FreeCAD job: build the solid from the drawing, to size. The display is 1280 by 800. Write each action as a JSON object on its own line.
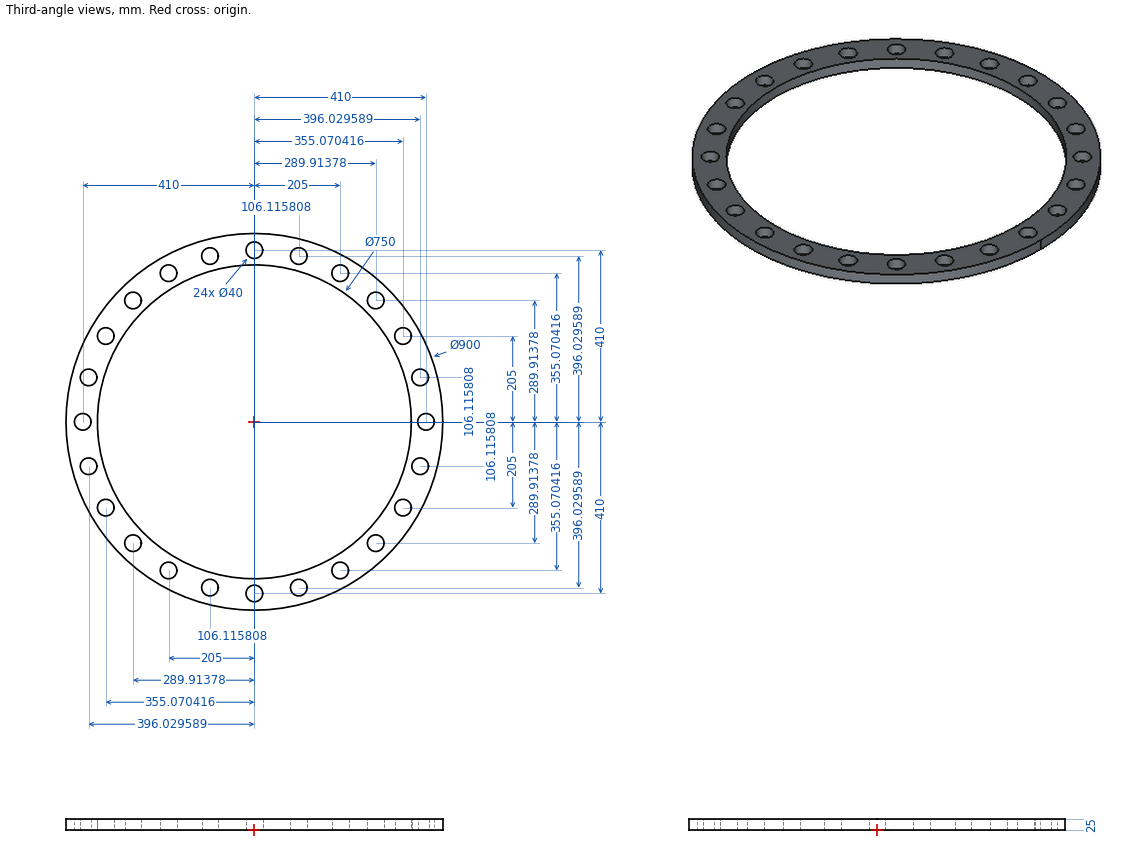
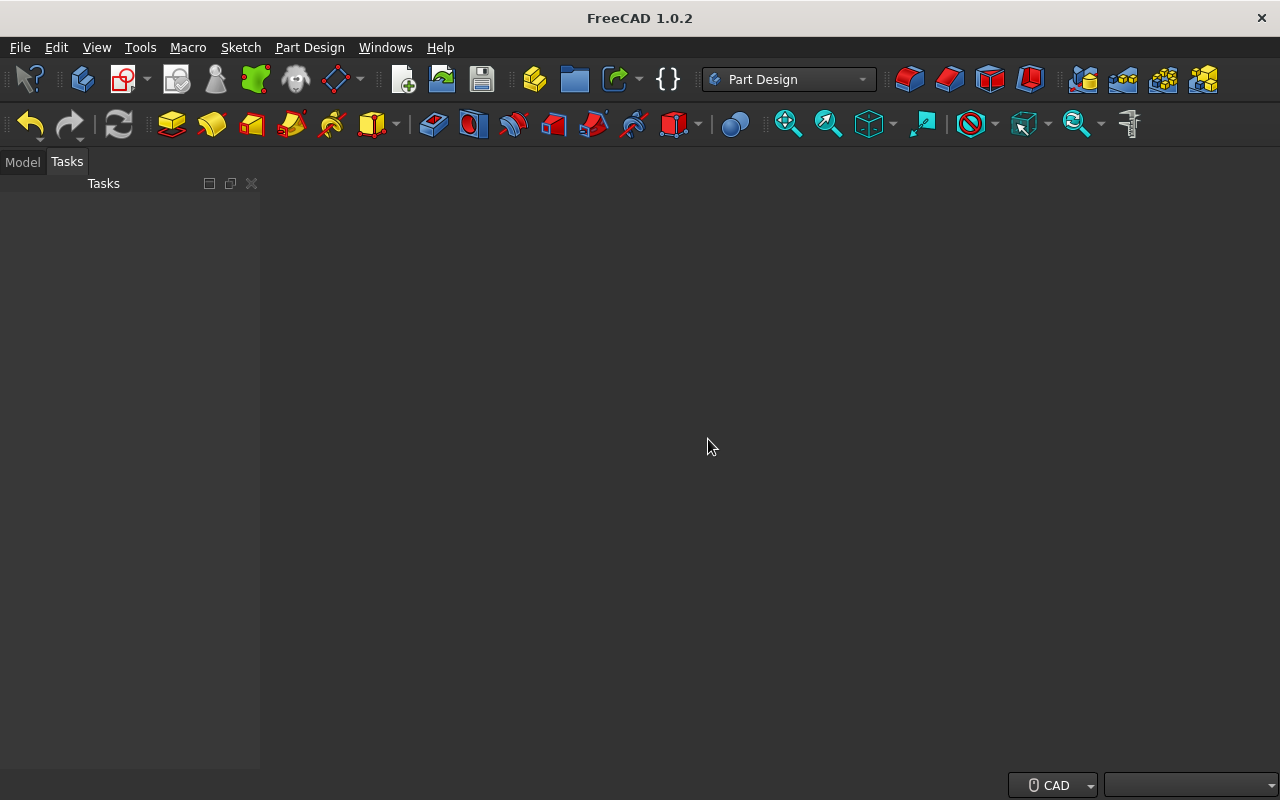
{"action": "left_click", "coordinate": [402, 80]}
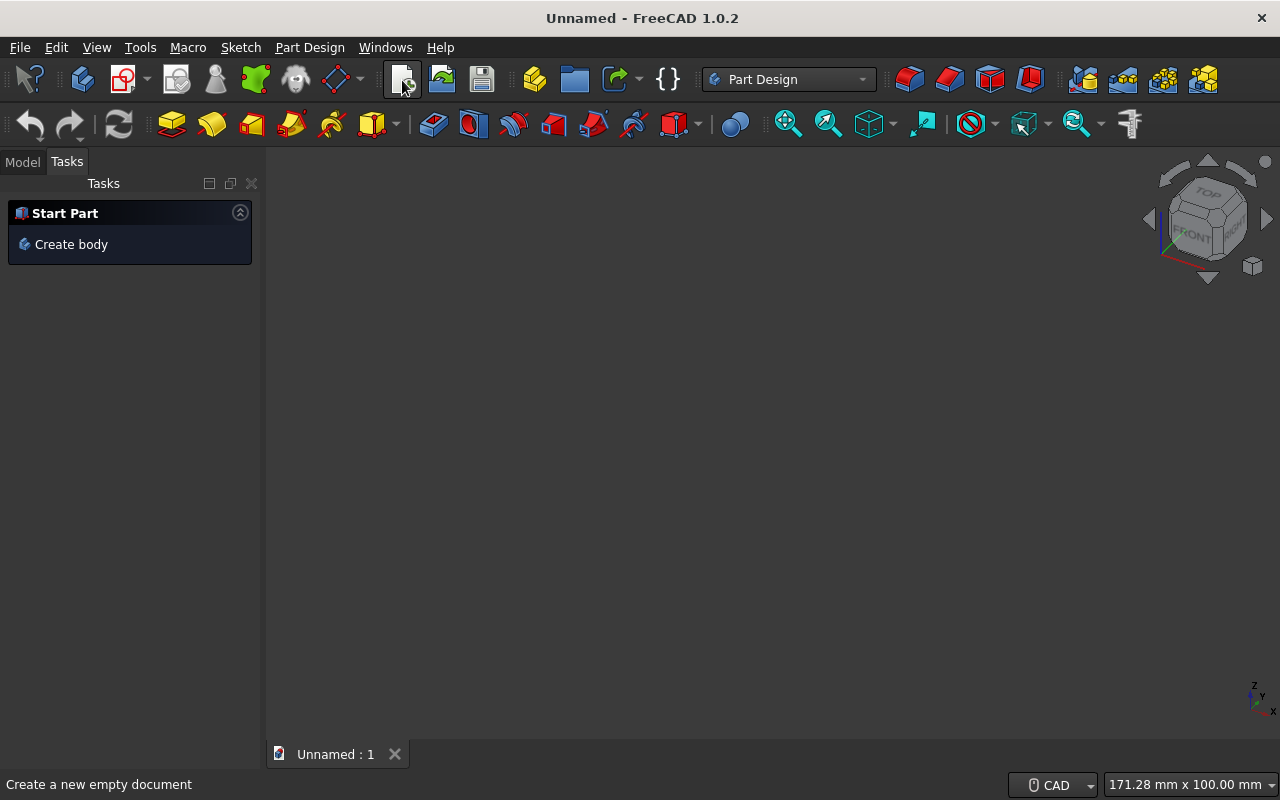
{"action": "left_click", "coordinate": [124, 80]}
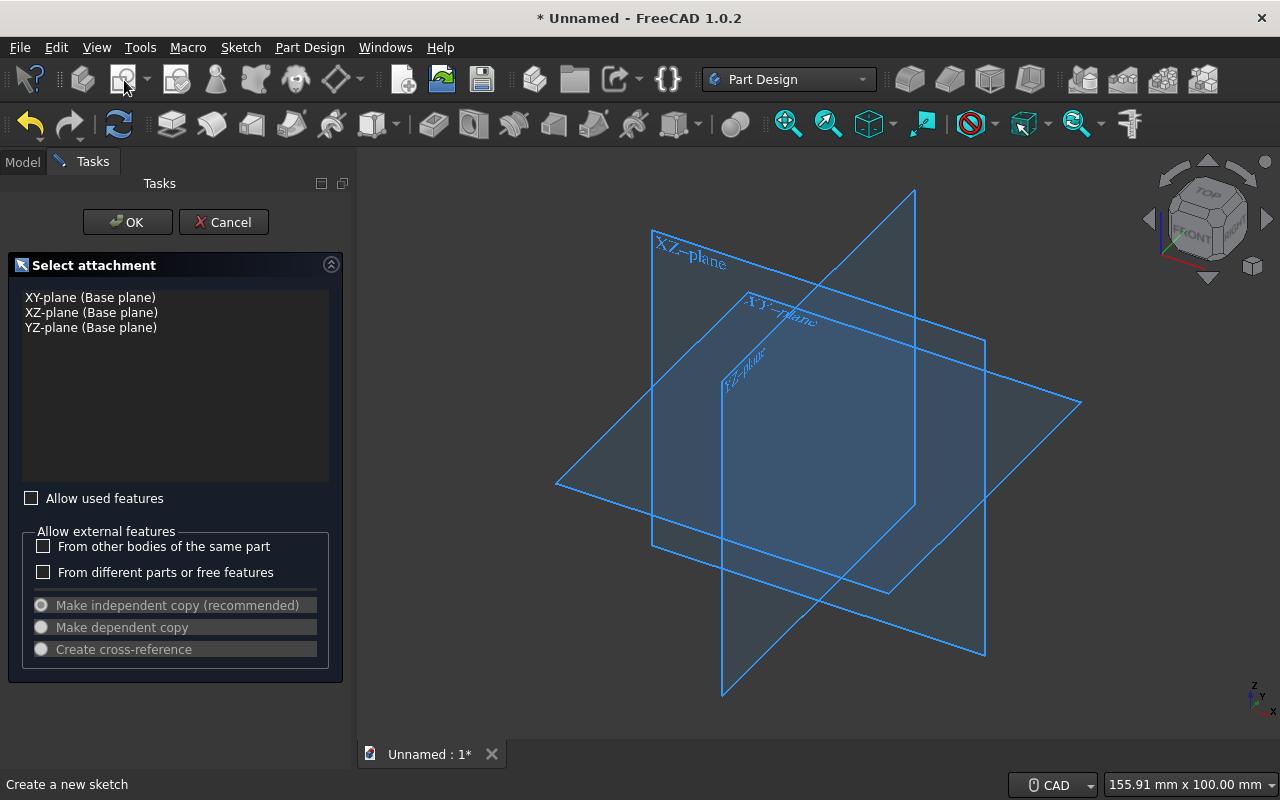
{"action": "left_click", "coordinate": [82, 298]}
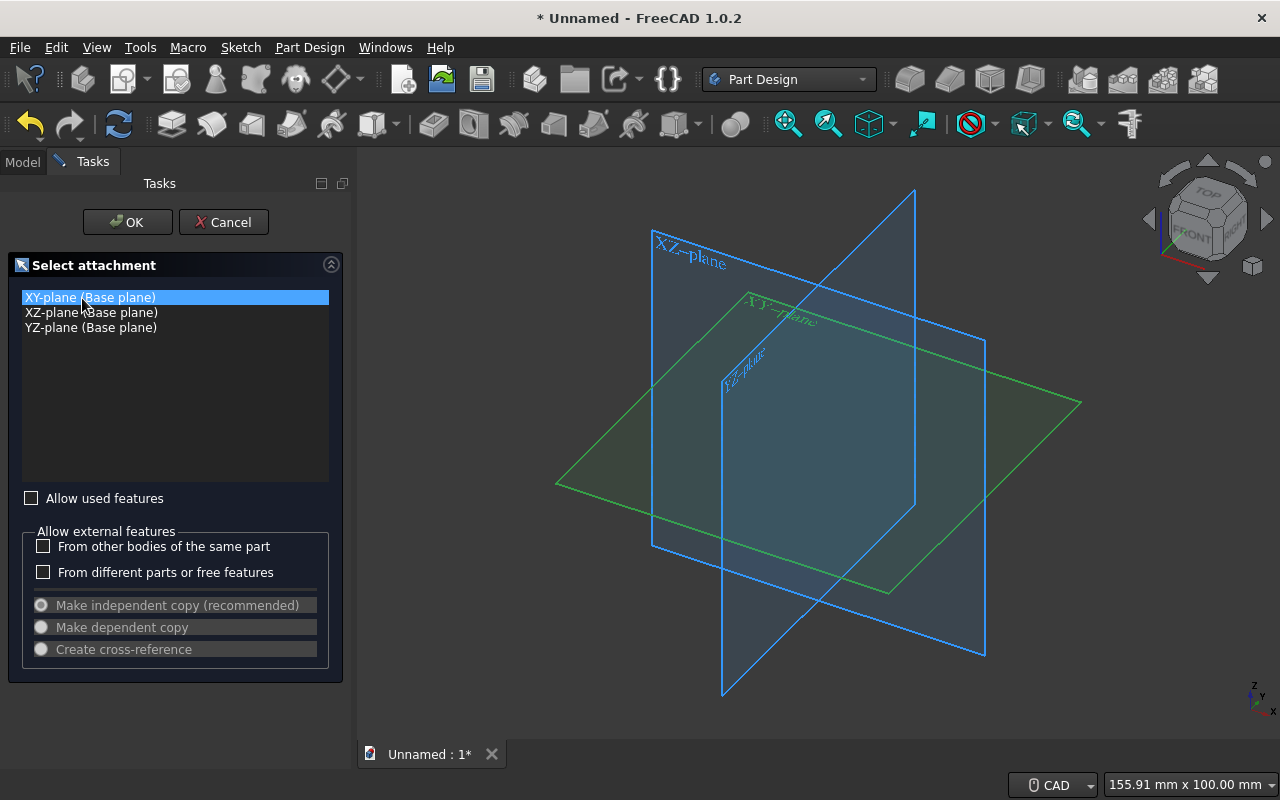
{"action": "left_click", "coordinate": [128, 222]}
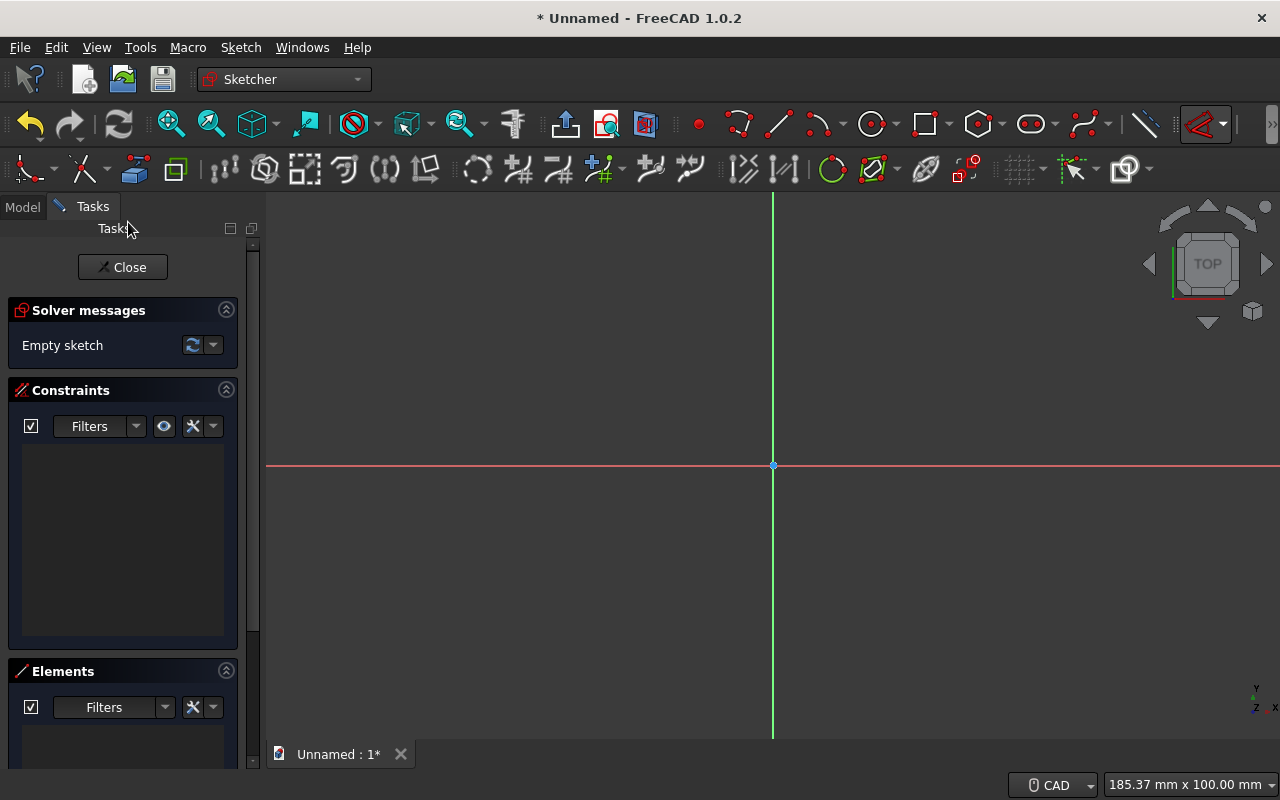
{"action": "scroll", "coordinate": [699, 466], "scroll_direction": "down", "scroll_amount": 13}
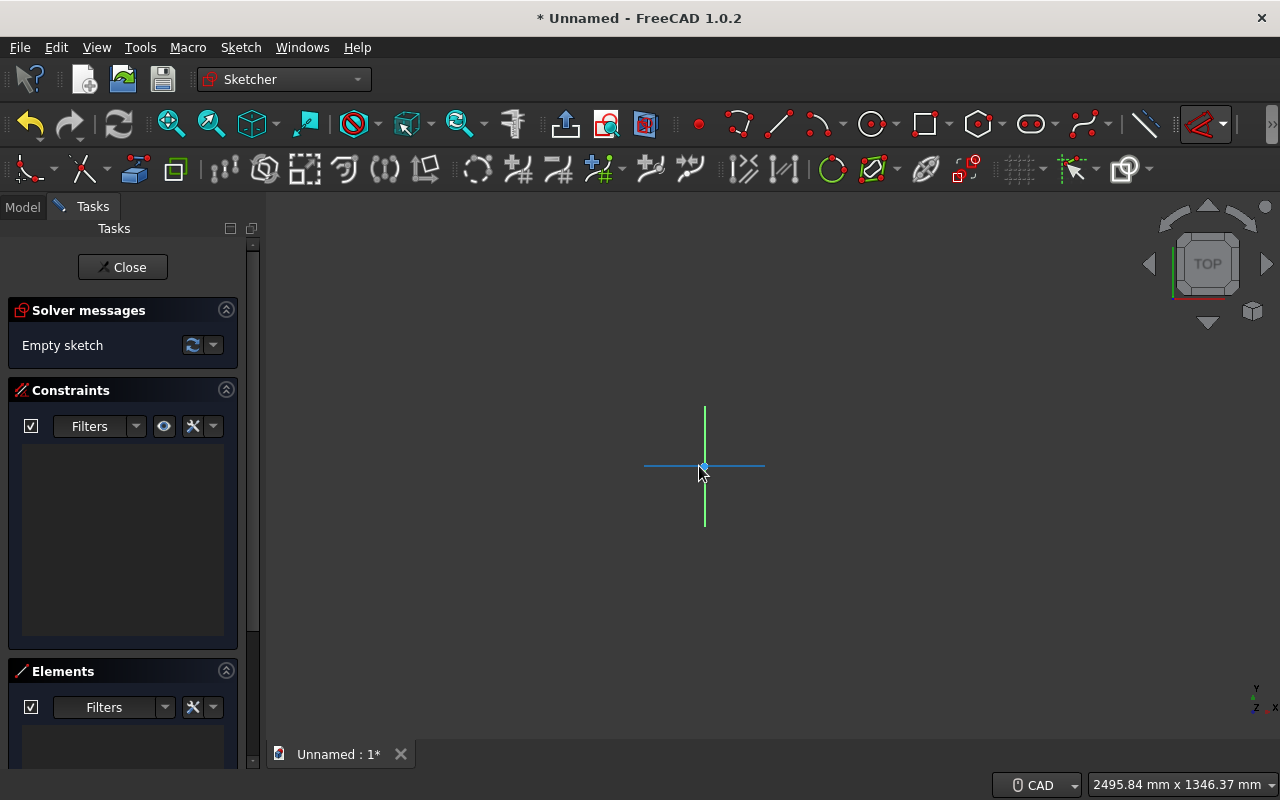
{"action": "left_click", "coordinate": [872, 124]}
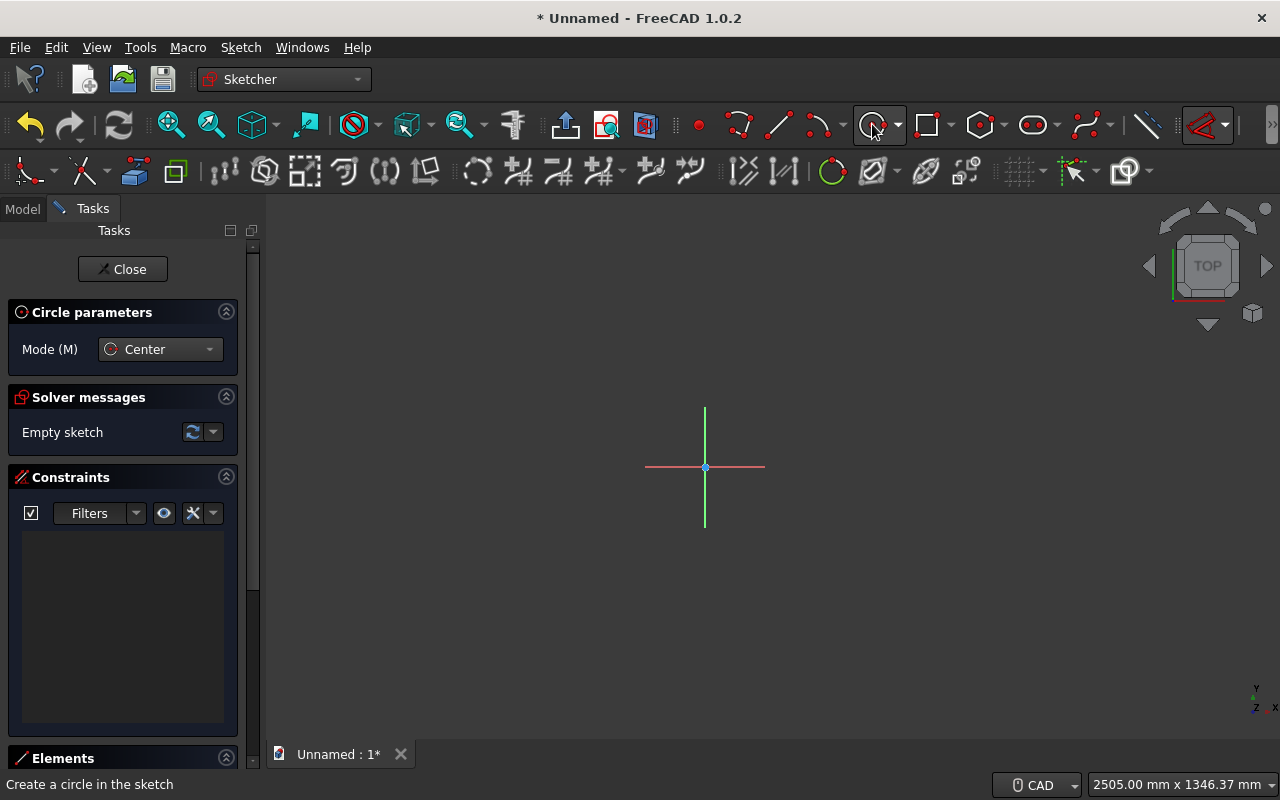
{"action": "left_click", "coordinate": [705, 467]}
{"action": "mouse_move", "coordinate": [834, 339]}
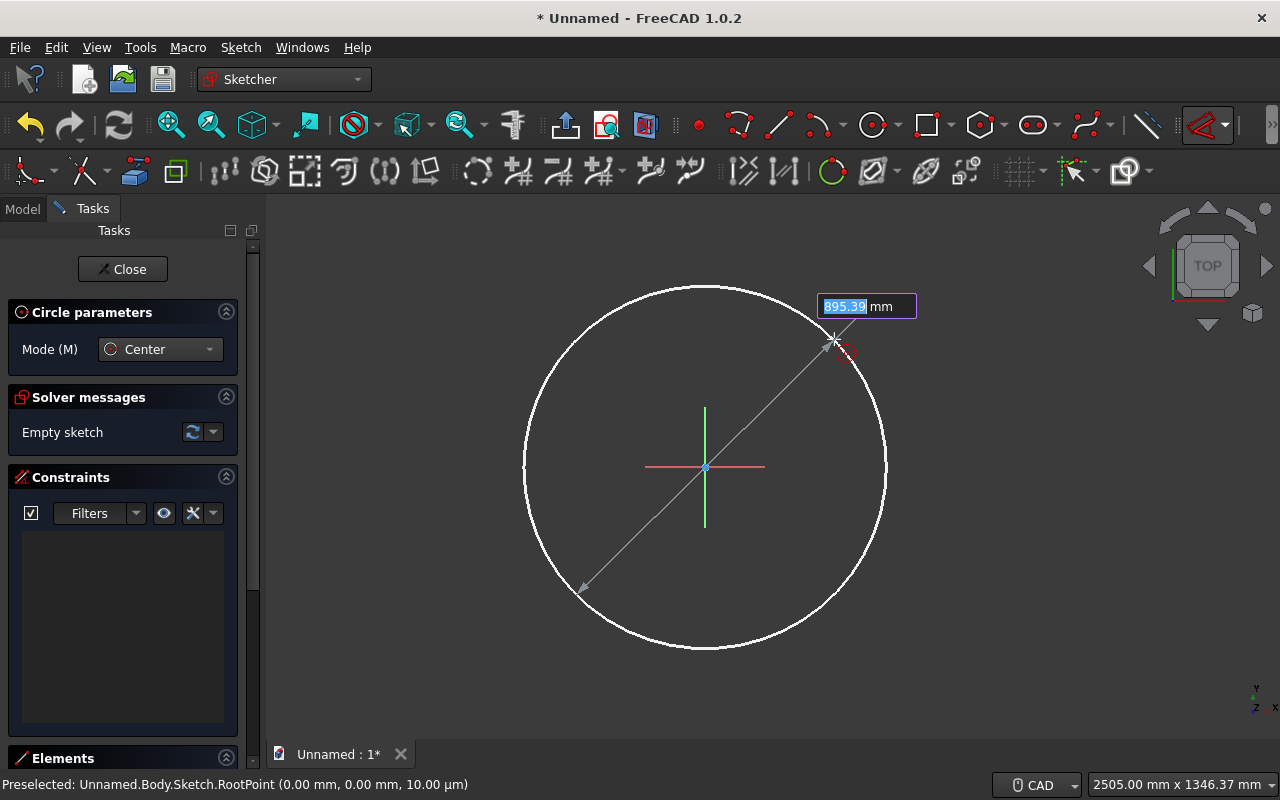
{"action": "type", "text": "900"}
{"action": "key", "text": "Return"}
{"action": "key", "text": "Escape"}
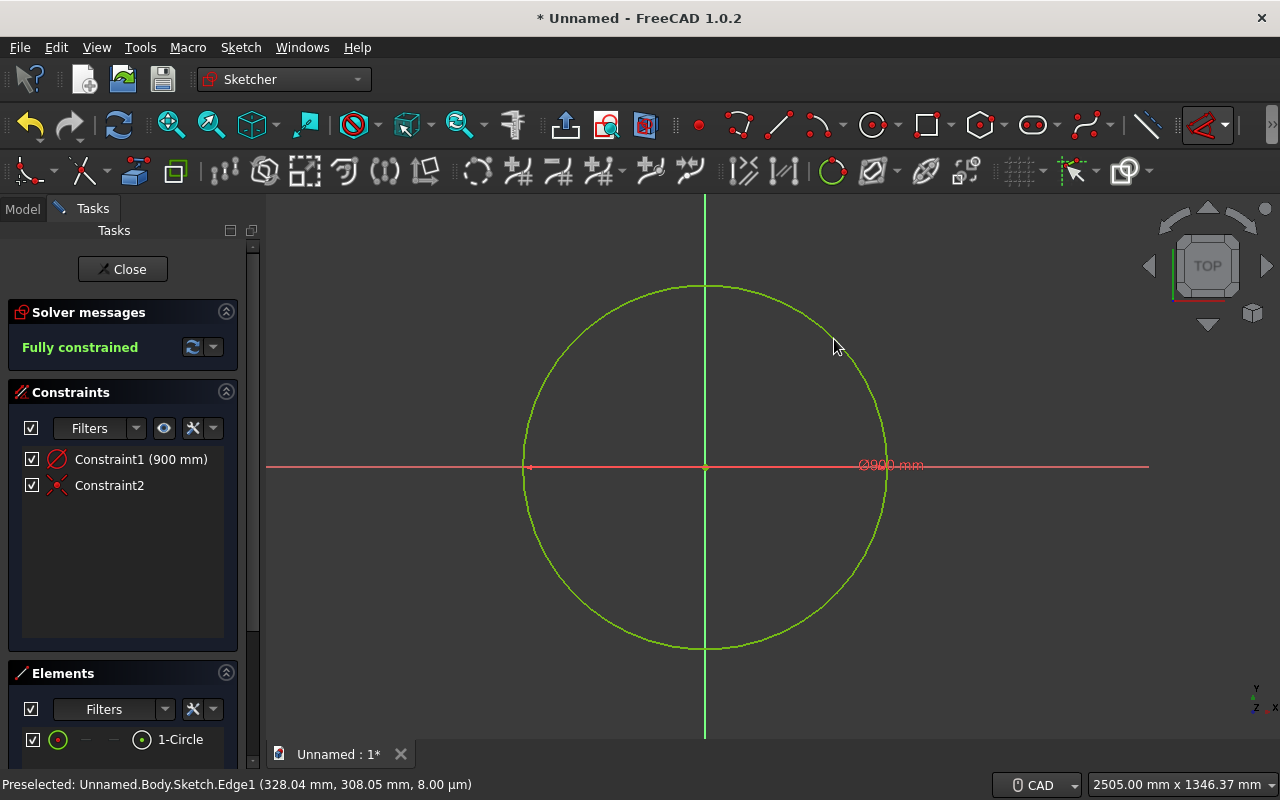
{"action": "left_click", "coordinate": [123, 269]}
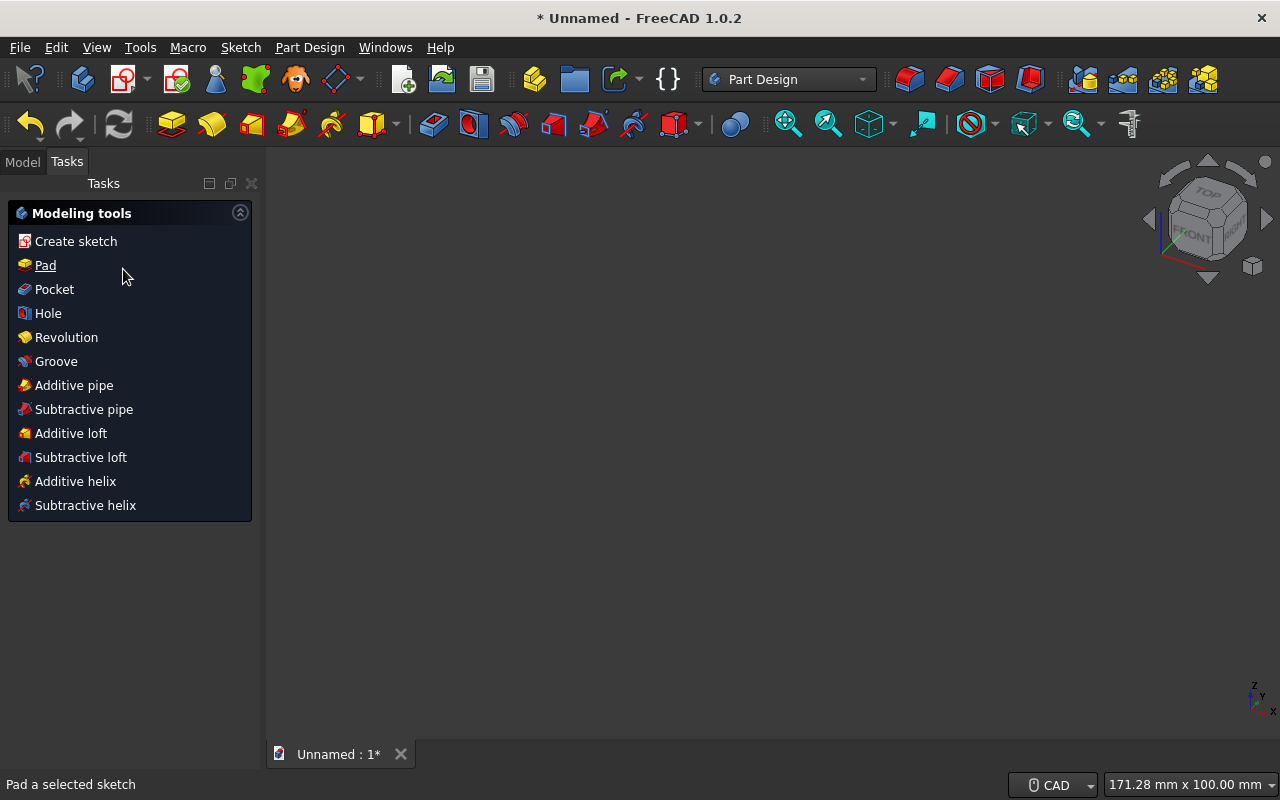
{"action": "left_click", "coordinate": [172, 124]}